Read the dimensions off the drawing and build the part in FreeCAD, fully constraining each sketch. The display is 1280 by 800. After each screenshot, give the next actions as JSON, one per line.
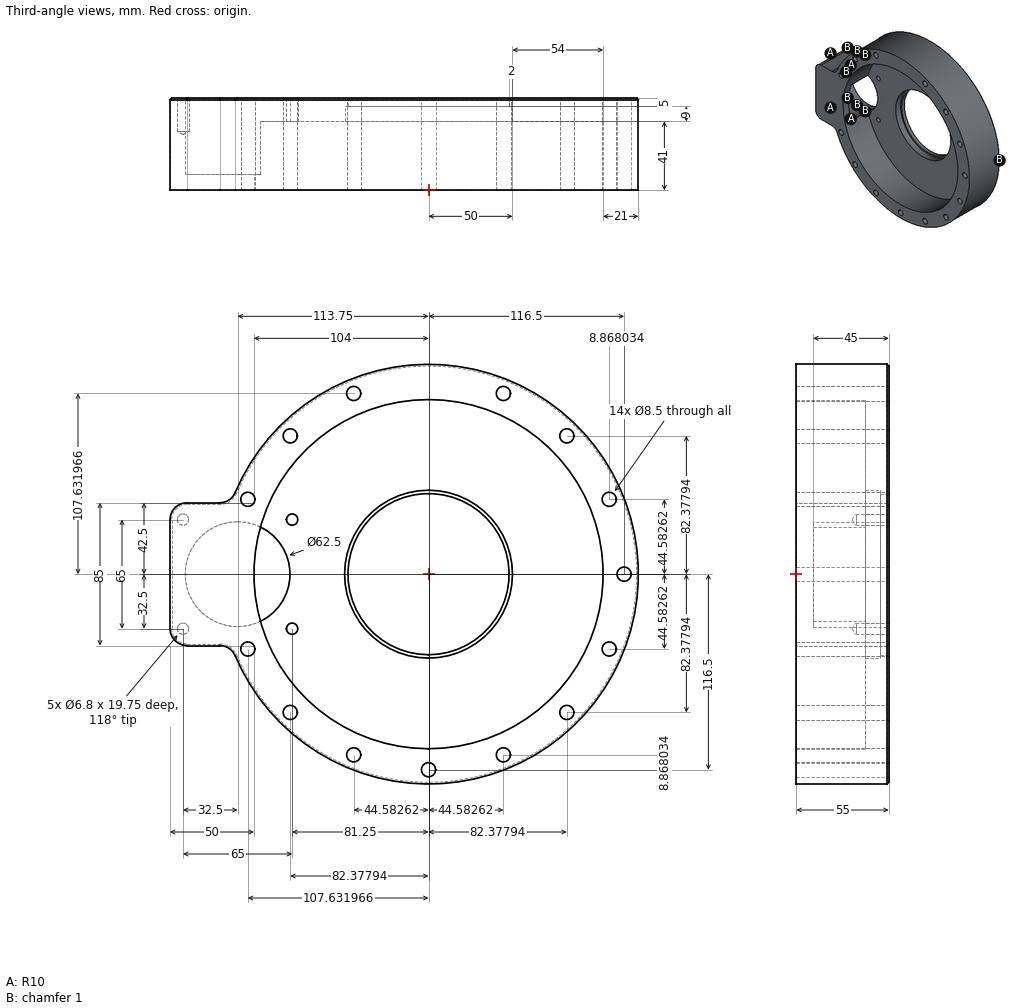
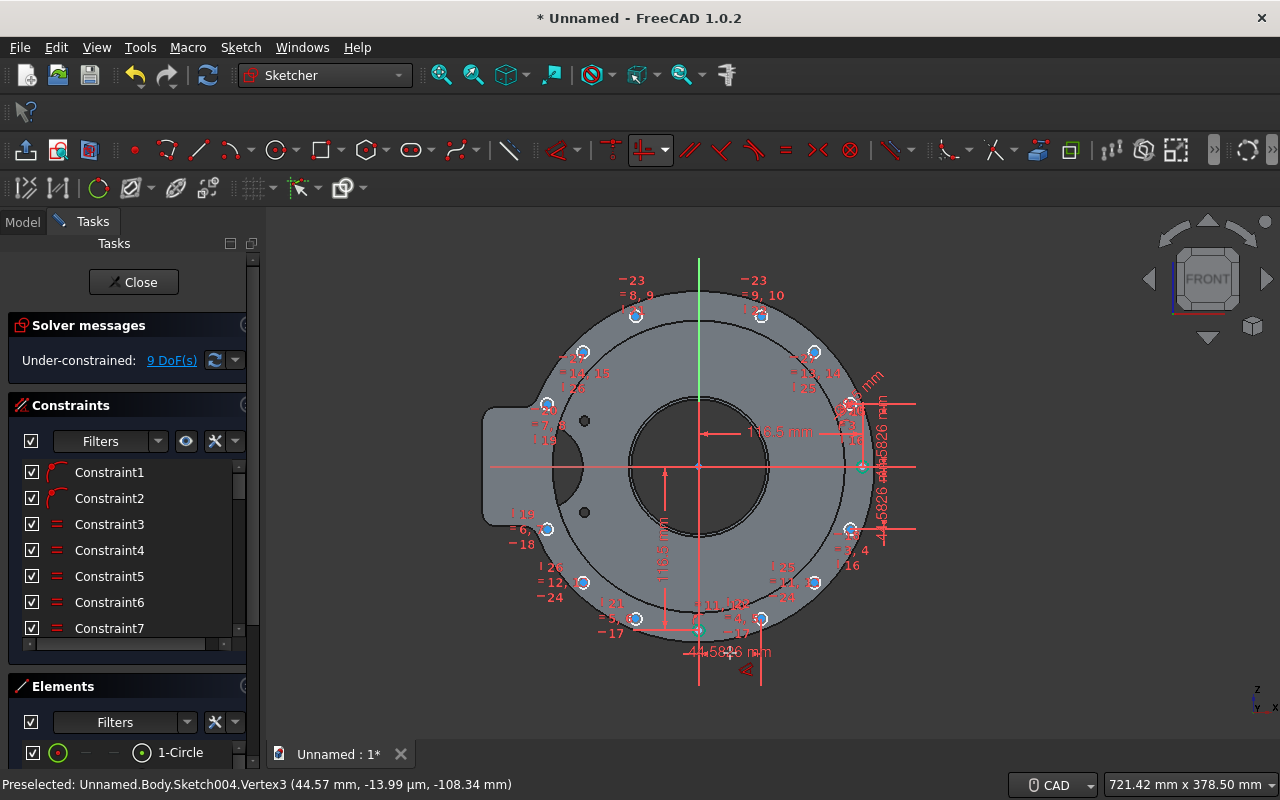
{"action": "left_click", "coordinate": [636, 619]}
{"action": "left_click", "coordinate": [653, 653]}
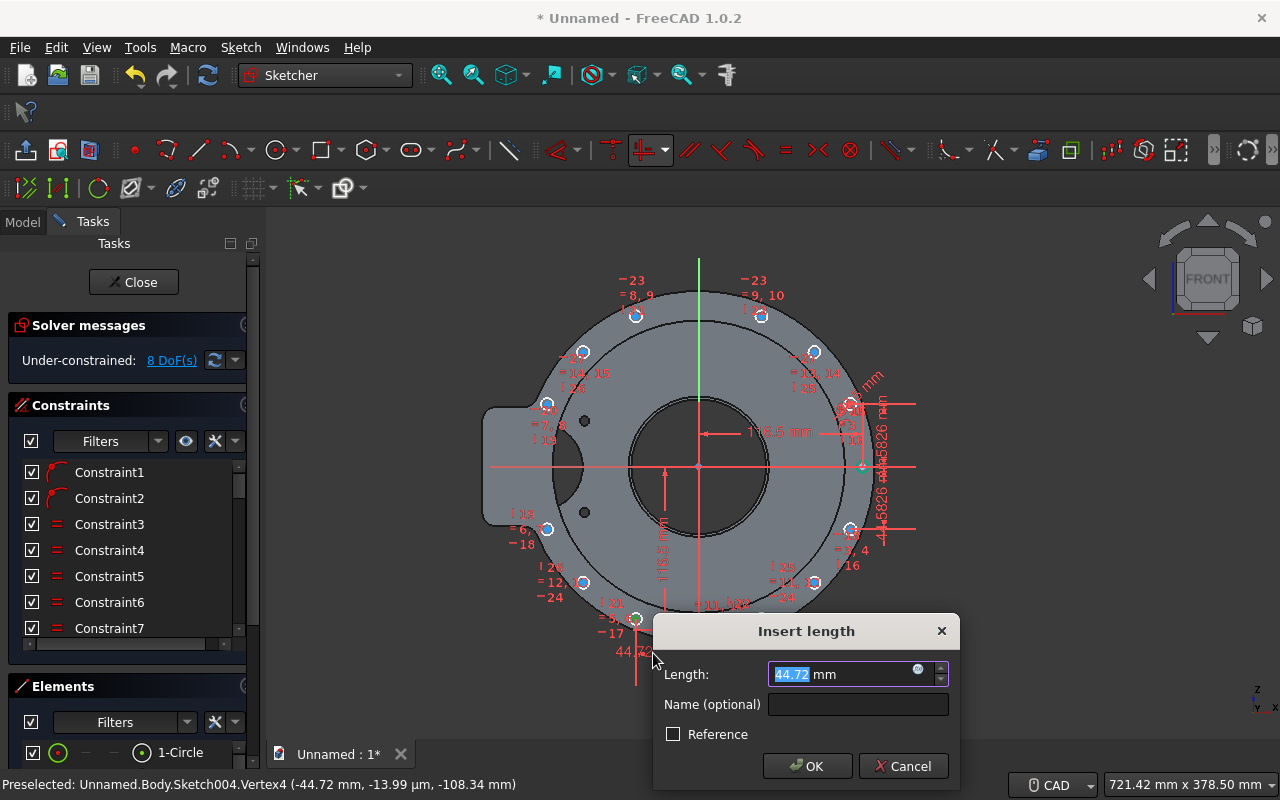
{"action": "type", "text": "44.58262"}
{"action": "key", "text": "Return"}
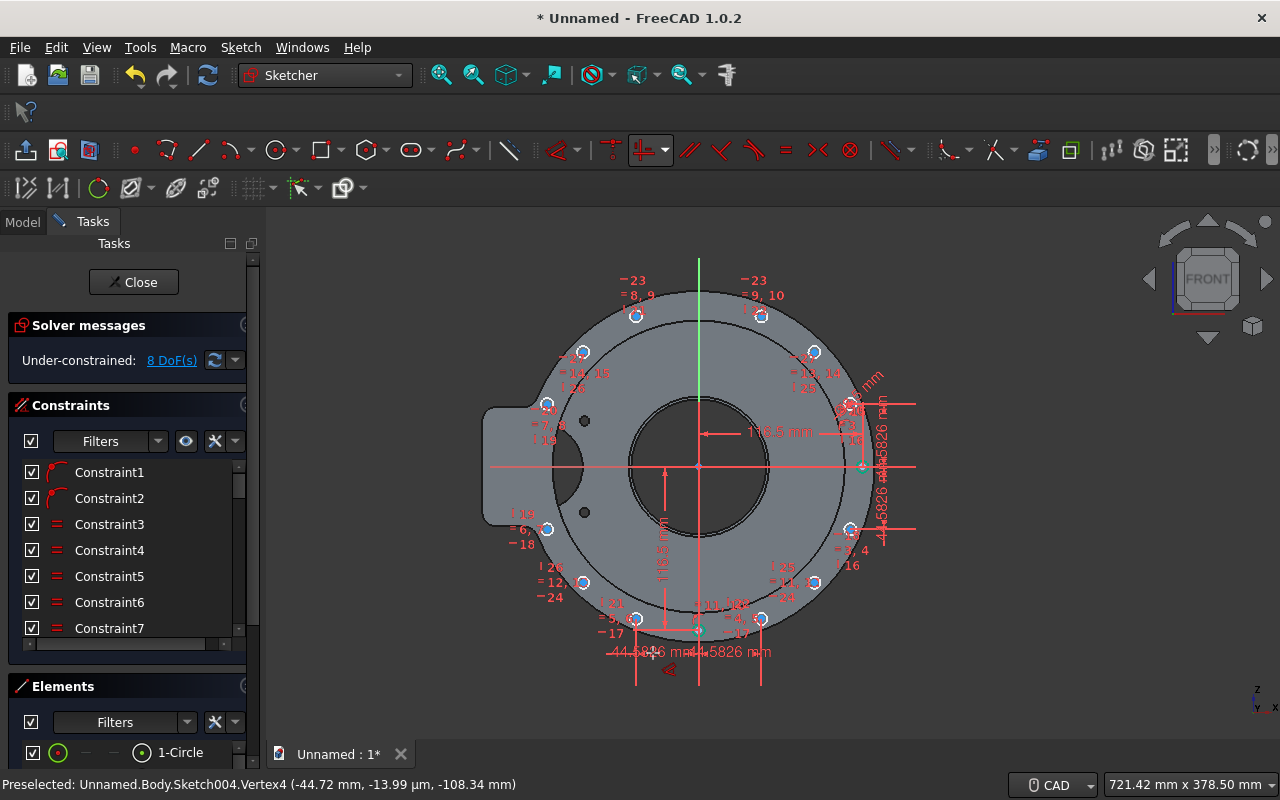
{"action": "left_click", "coordinate": [814, 583]}
{"action": "left_click", "coordinate": [730, 617]}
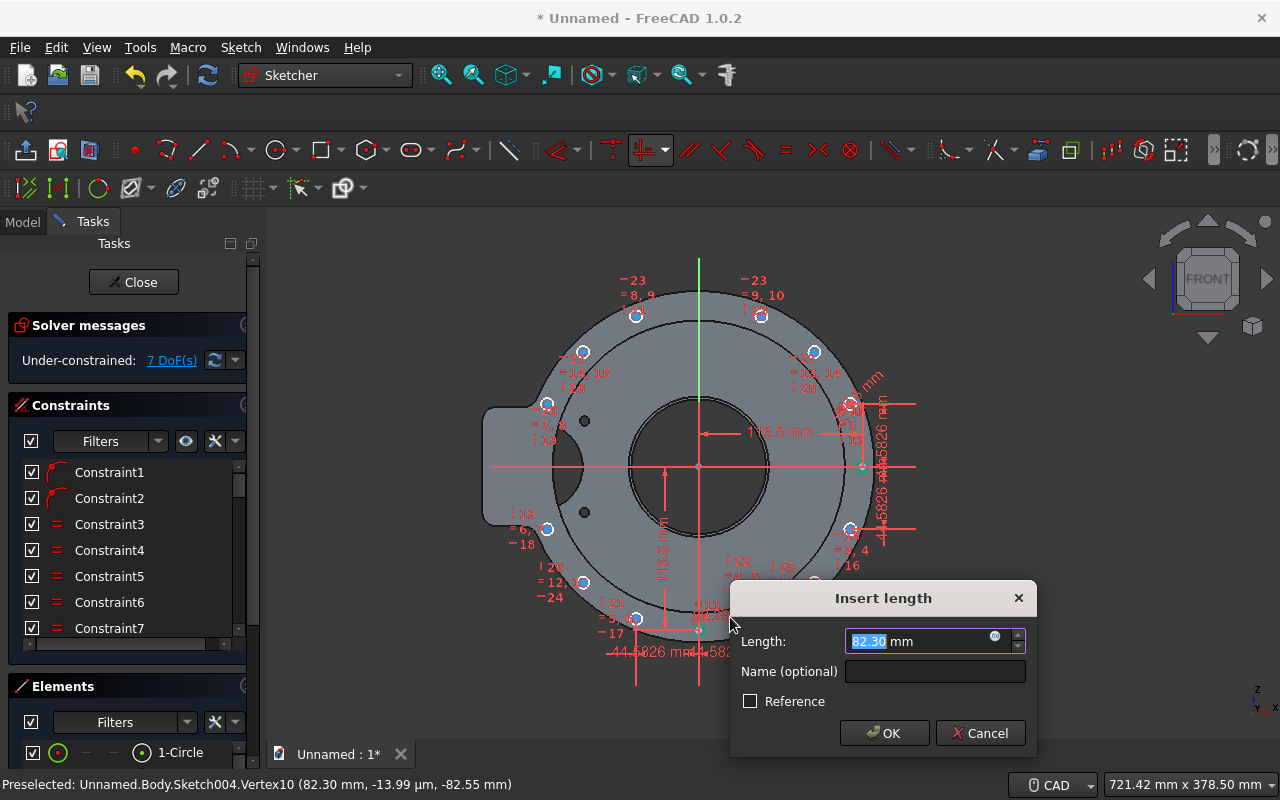
{"action": "type", "text": "82.37794"}
{"action": "key", "text": "Return"}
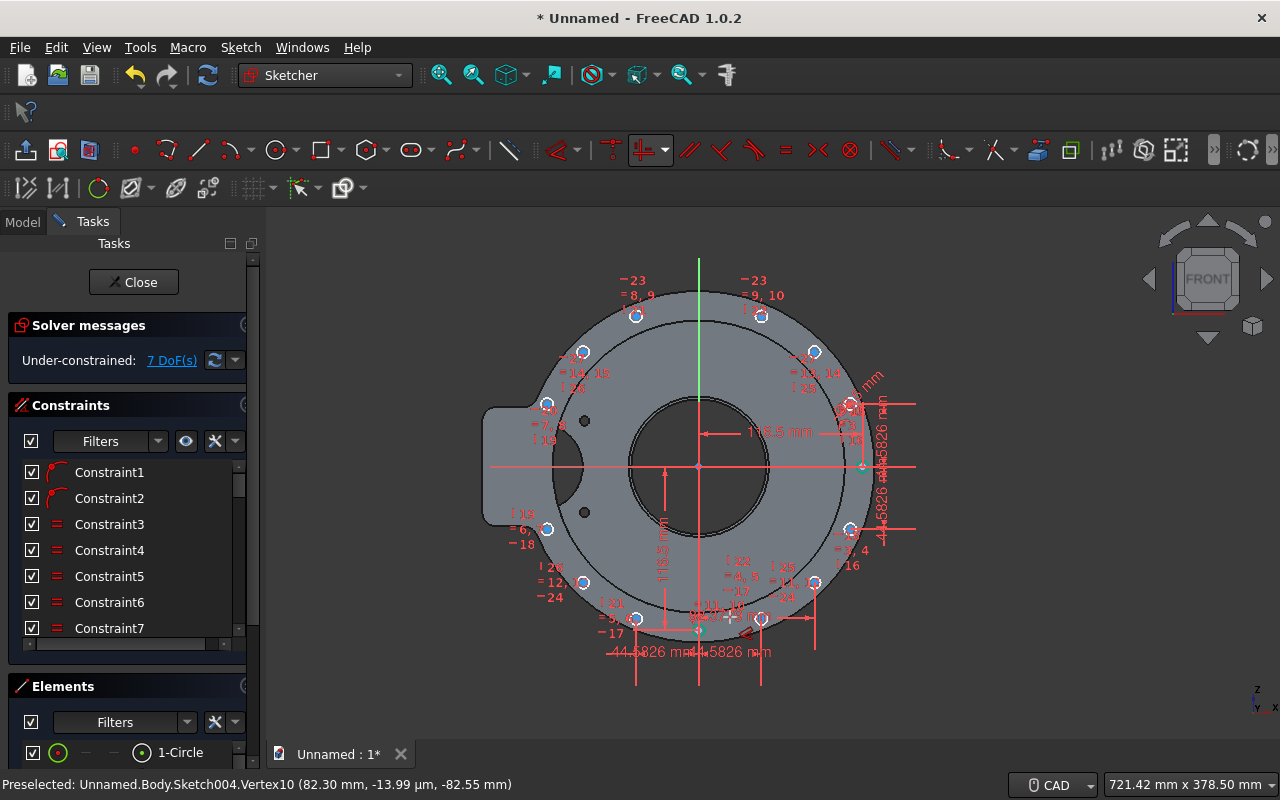
{"action": "left_click", "coordinate": [815, 583]}
{"action": "left_click", "coordinate": [849, 551]}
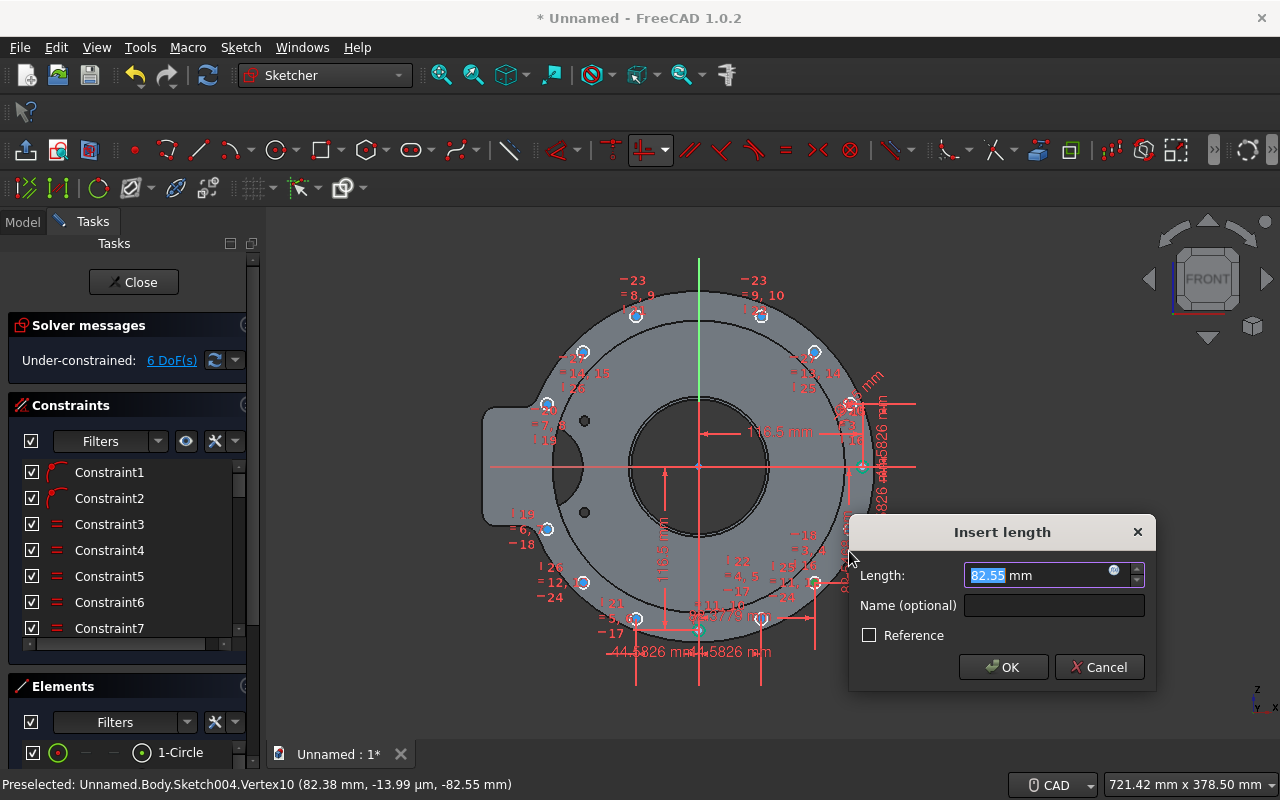
{"action": "type", "text": "82.37794"}
{"action": "key", "text": "Return"}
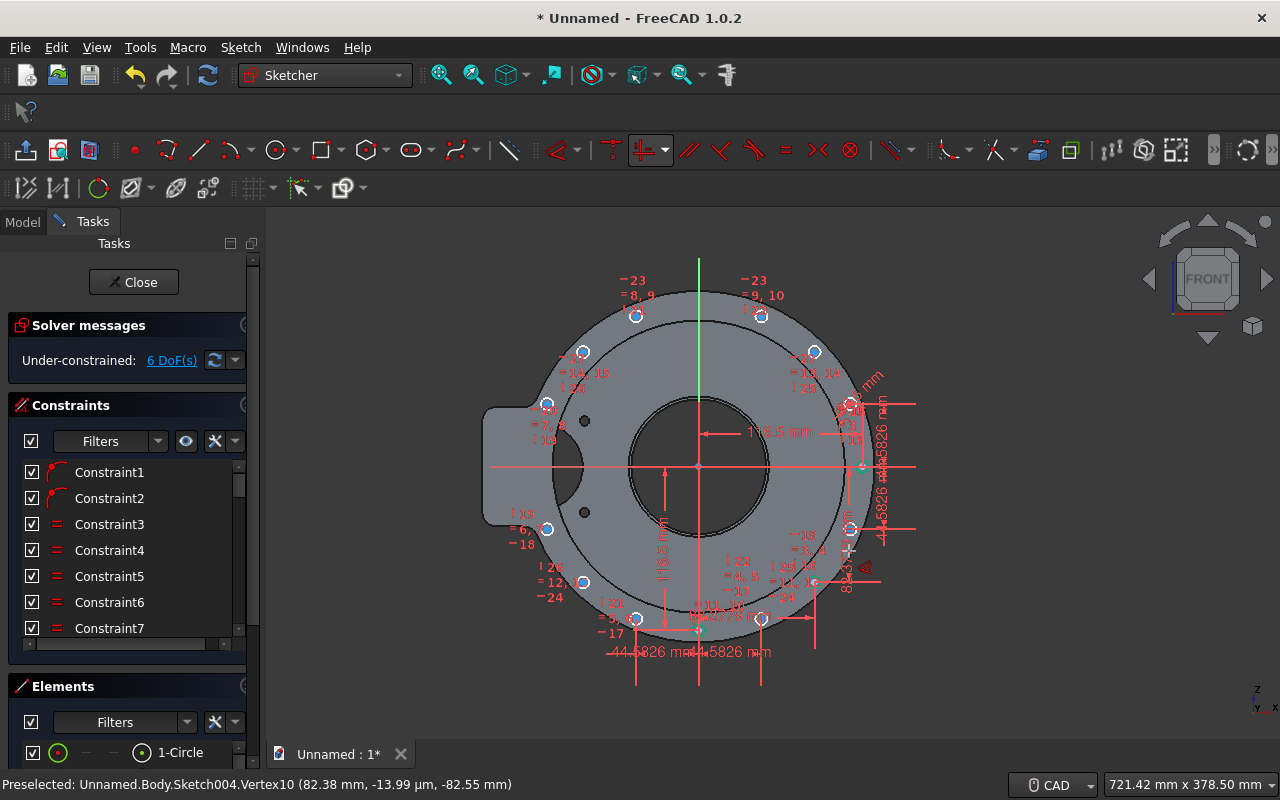
{"action": "left_click", "coordinate": [583, 582]}
{"action": "left_click", "coordinate": [614, 616]}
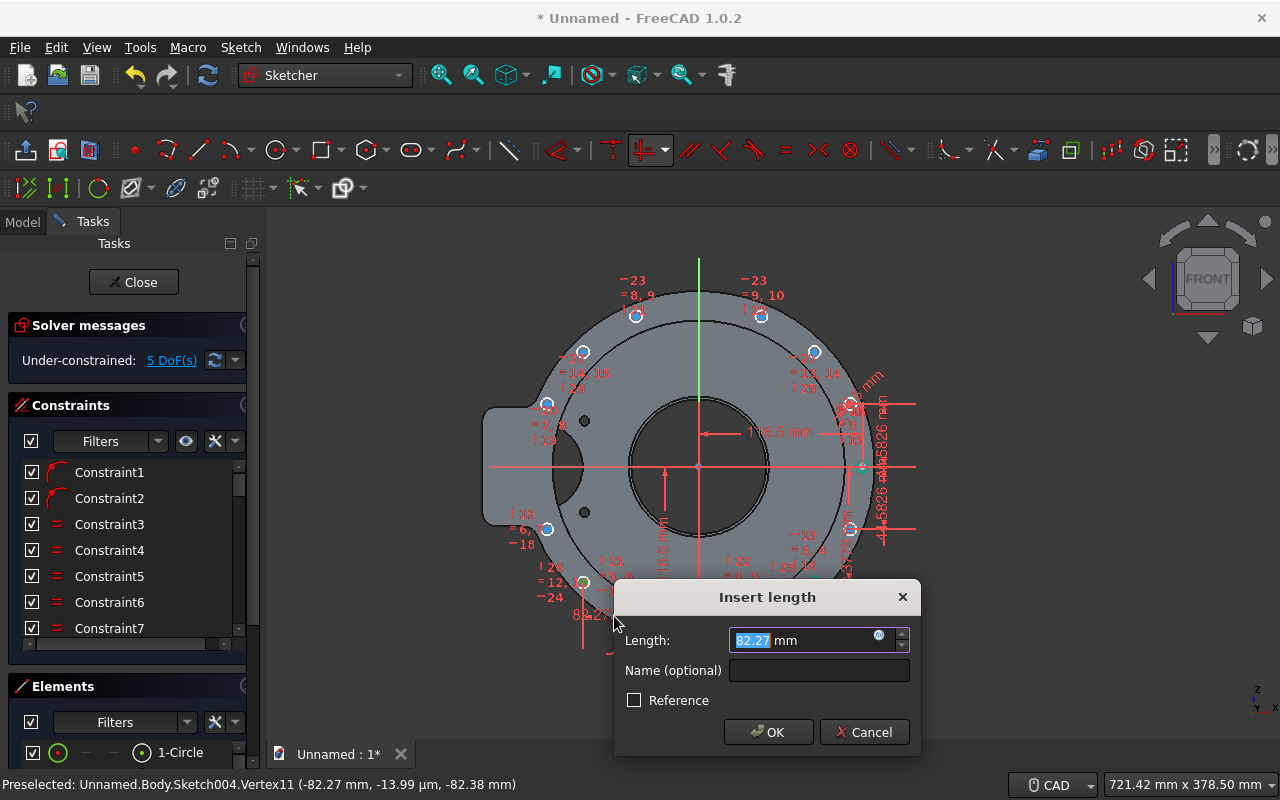
{"action": "type", "text": "82.37794"}
{"action": "key", "text": "Return"}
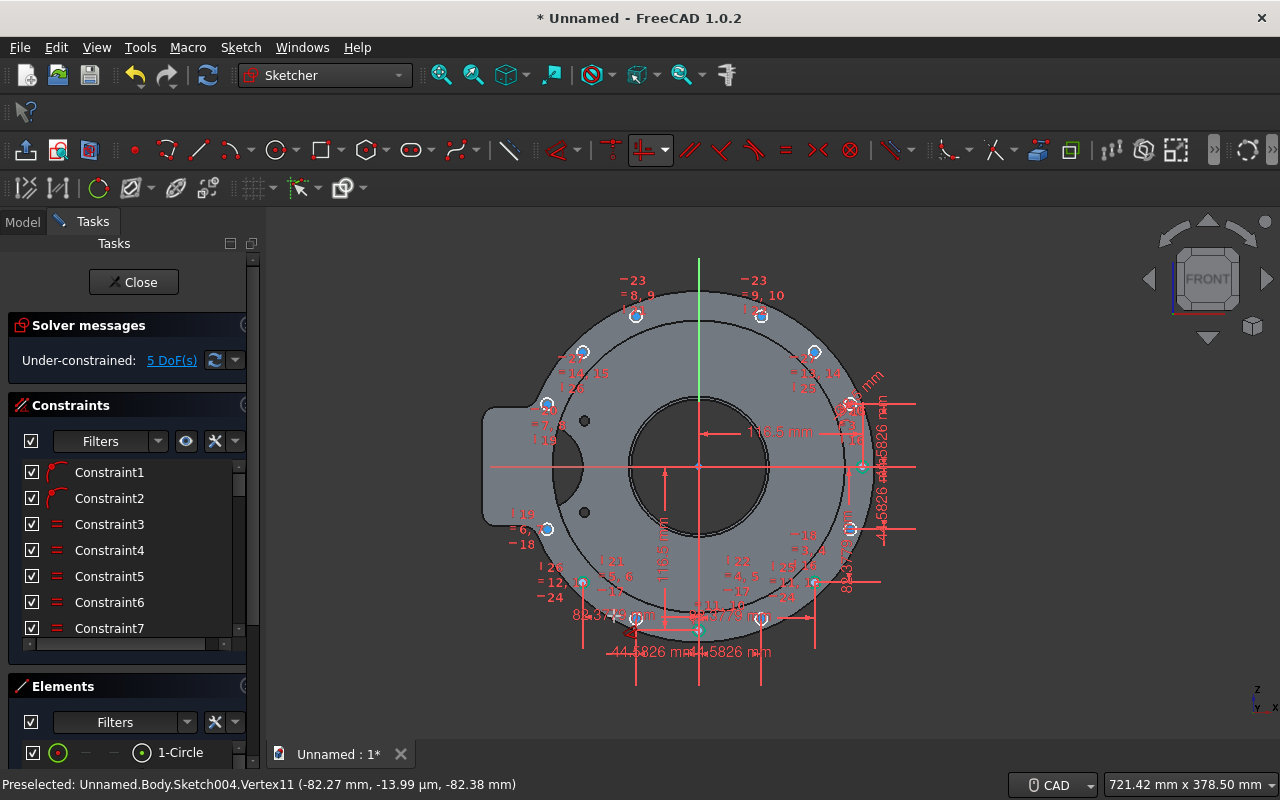
{"action": "left_click", "coordinate": [815, 352]}
{"action": "left_click", "coordinate": [849, 369]}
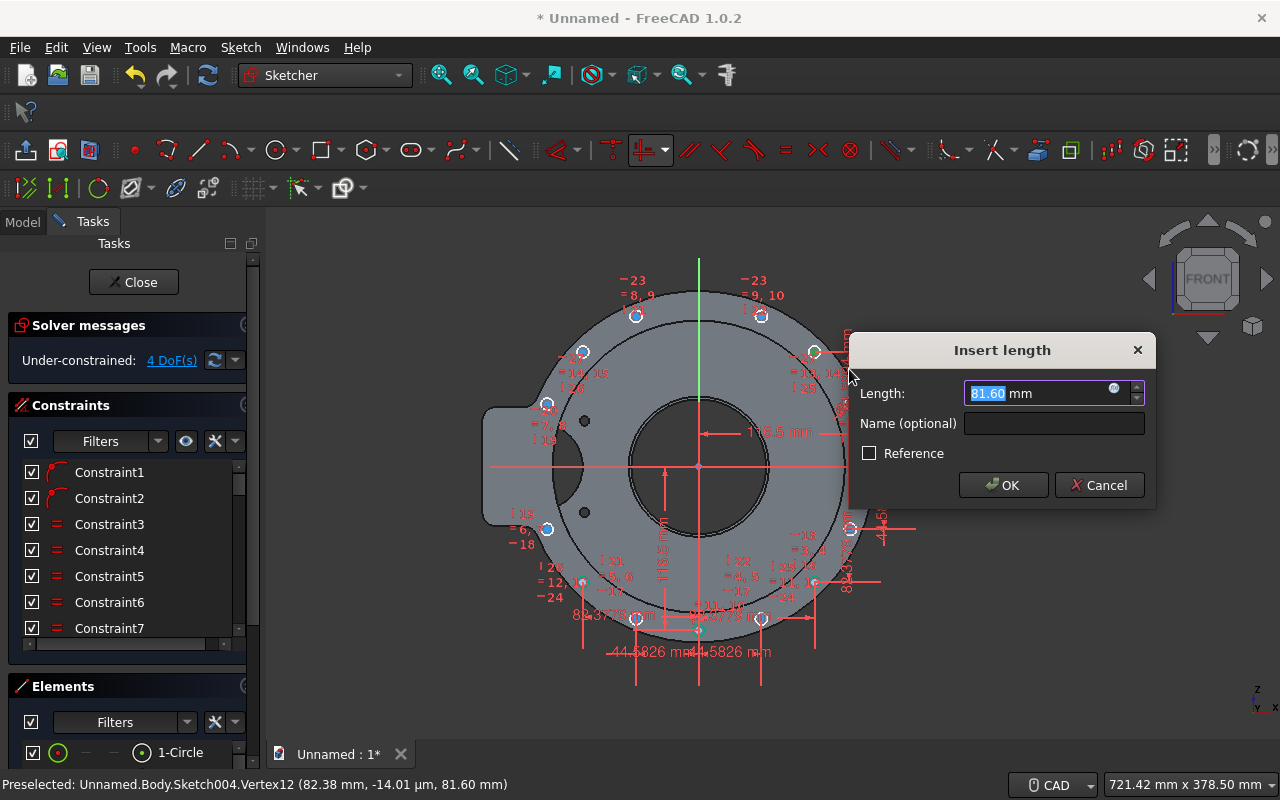
{"action": "type", "text": "82.37794"}
{"action": "key", "text": "Return"}